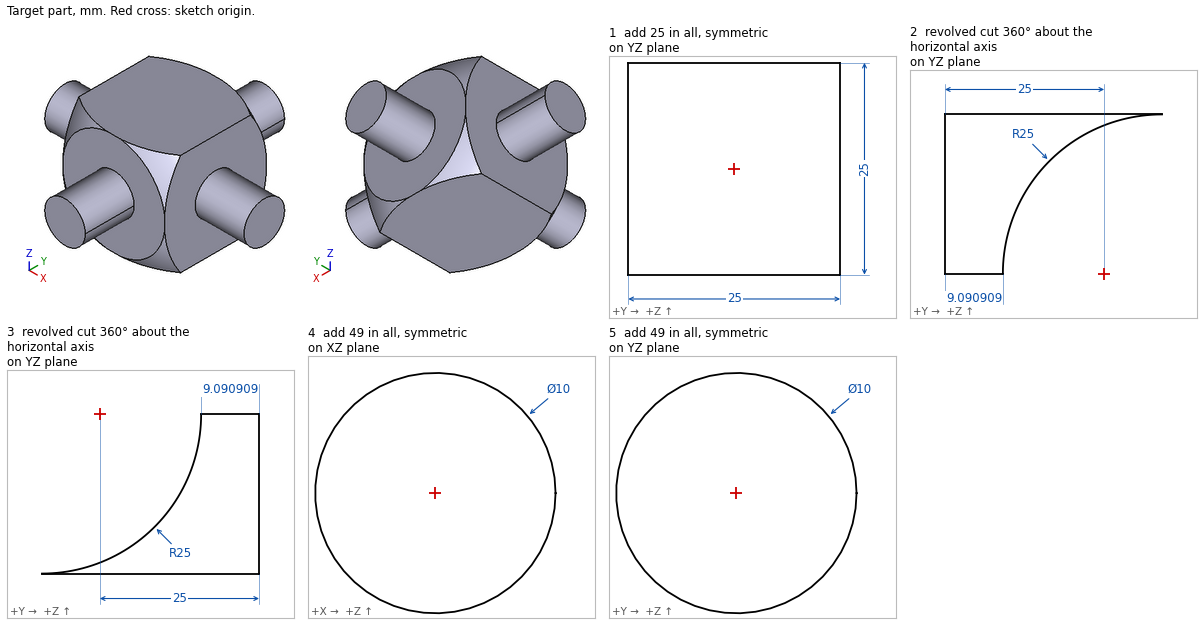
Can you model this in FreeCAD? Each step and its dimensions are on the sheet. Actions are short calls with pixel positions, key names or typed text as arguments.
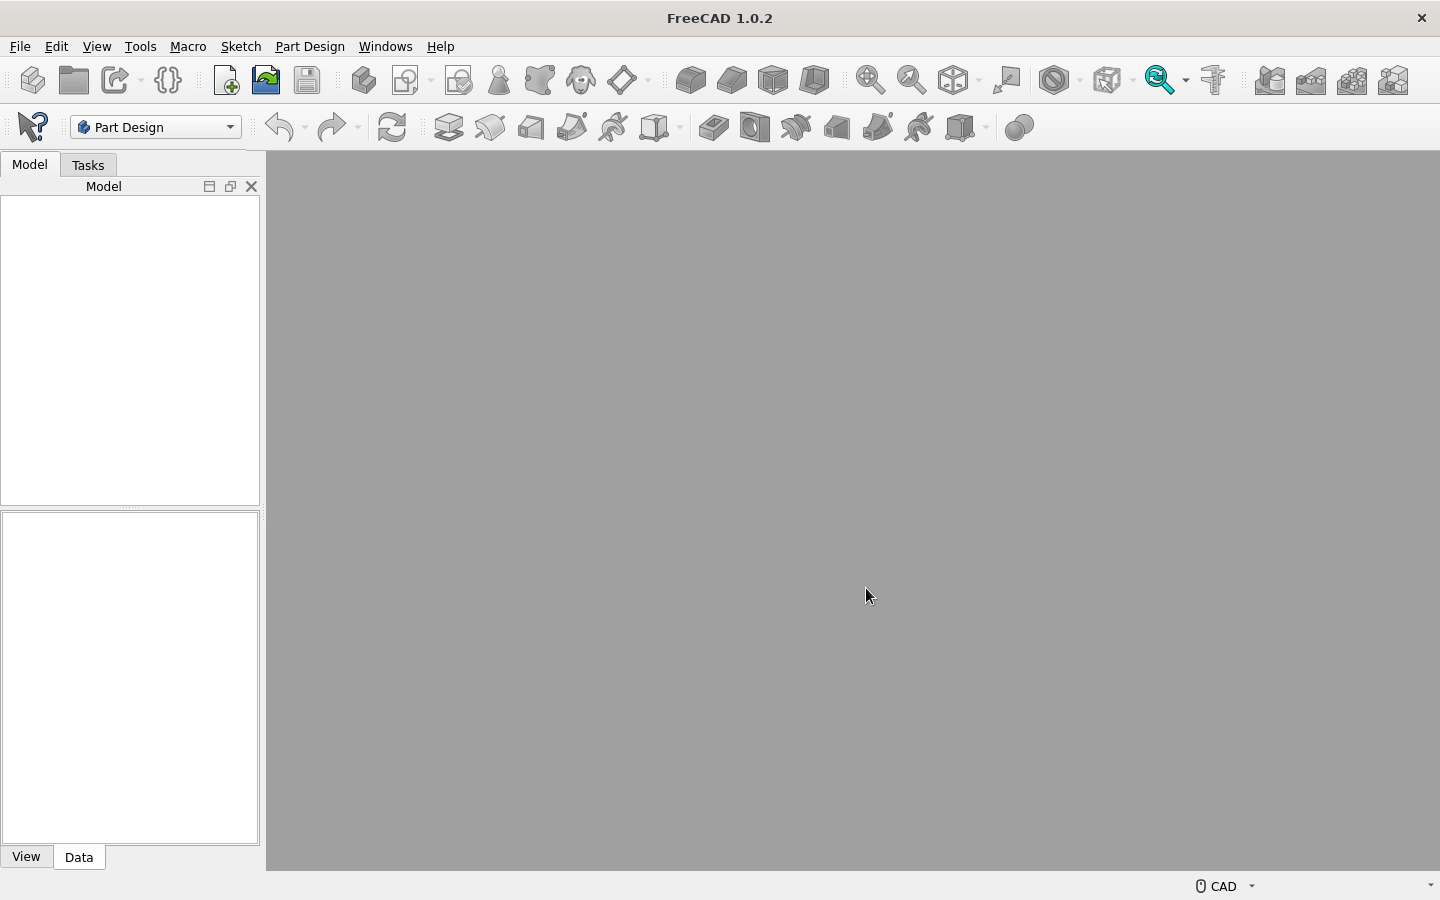
key(ctrl+n)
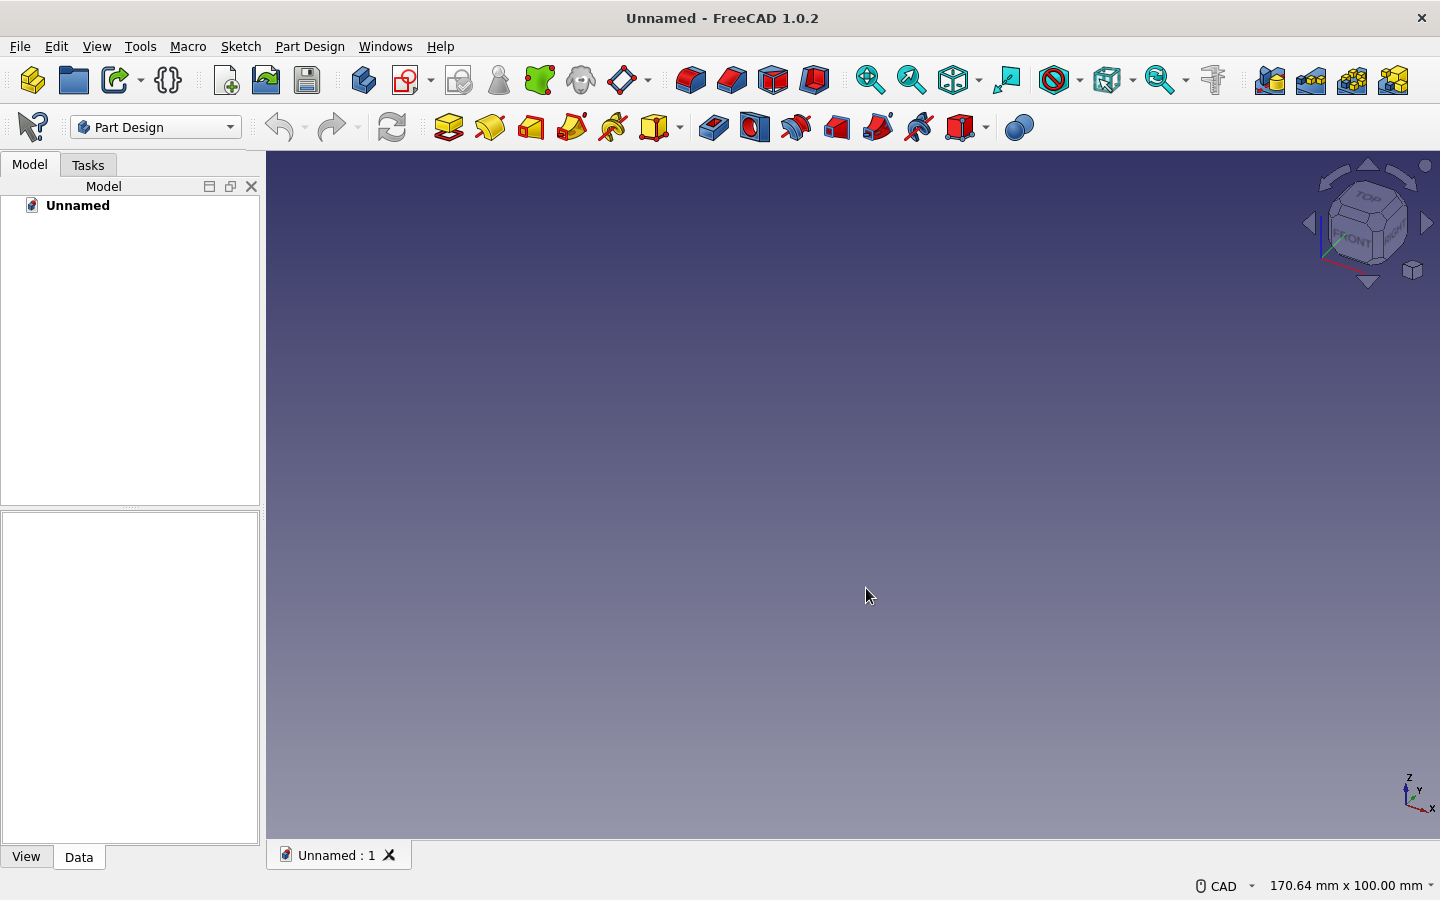
click(404, 80)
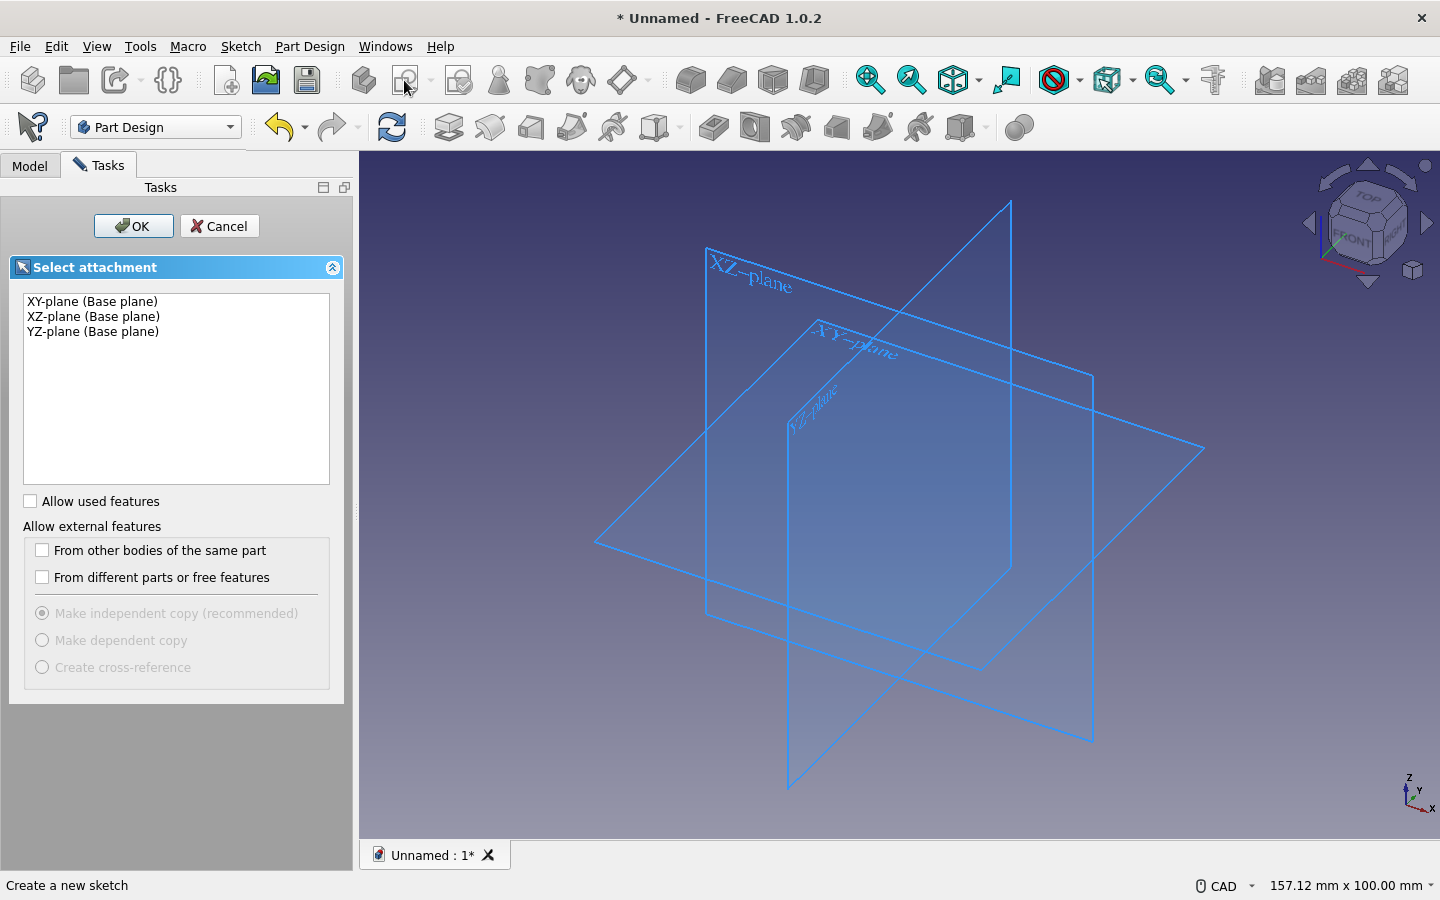
click(84, 332)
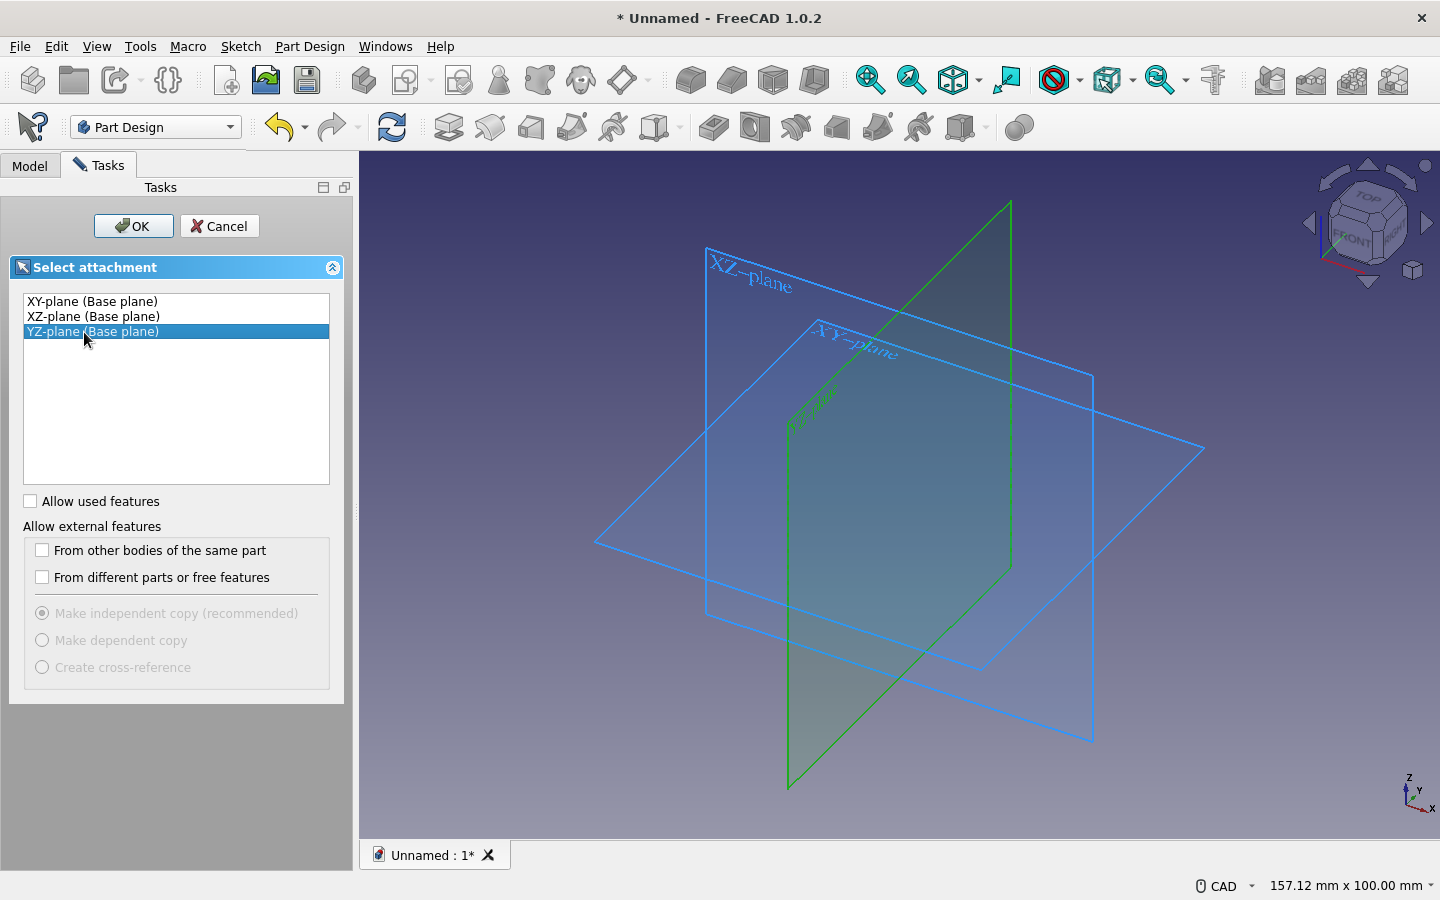
click(134, 226)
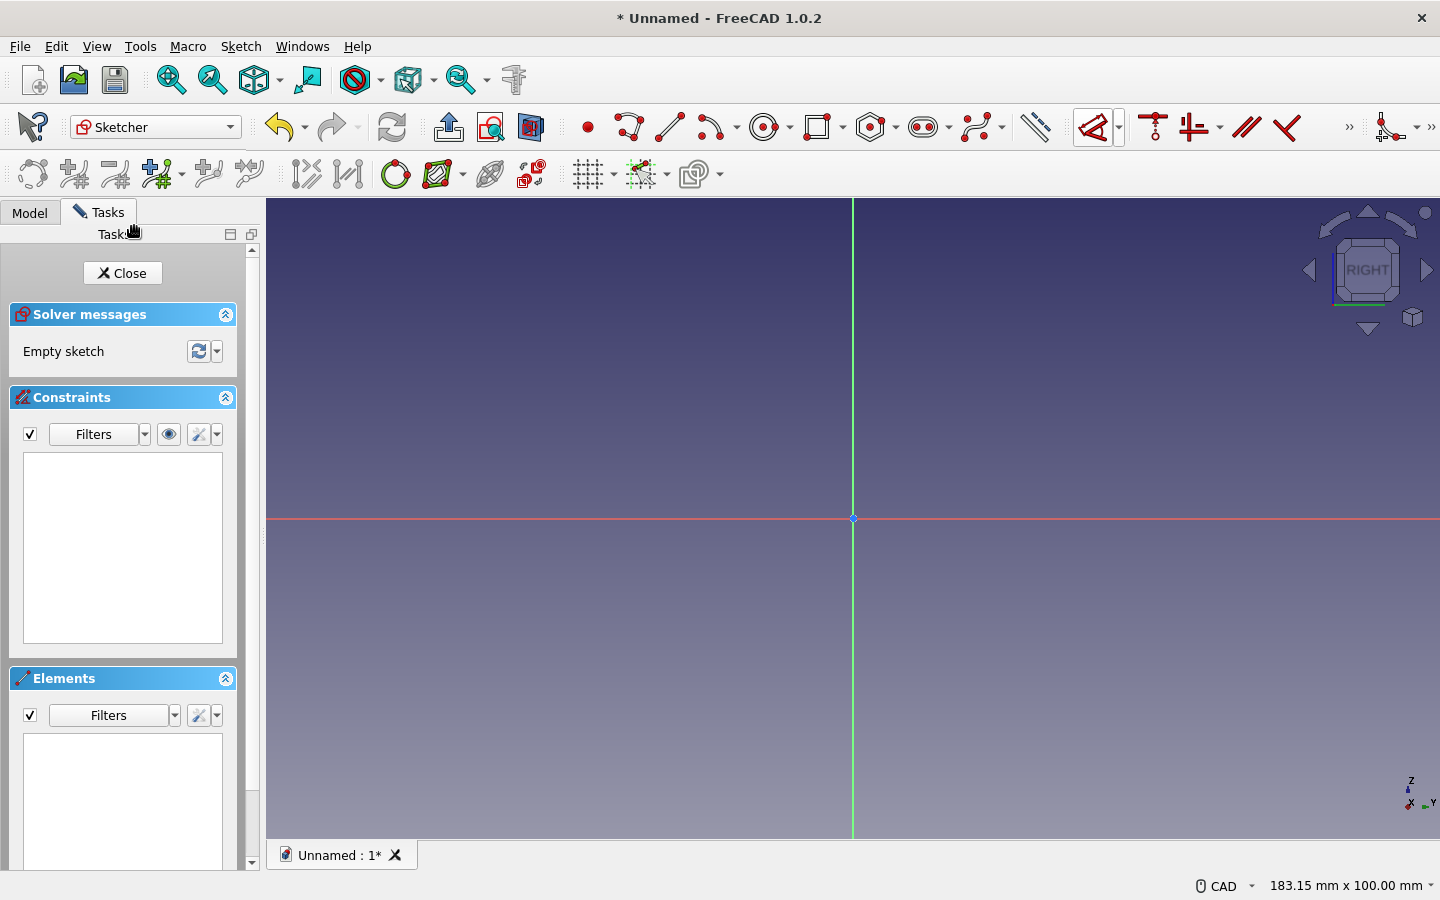
scroll(893, 518, up, 5)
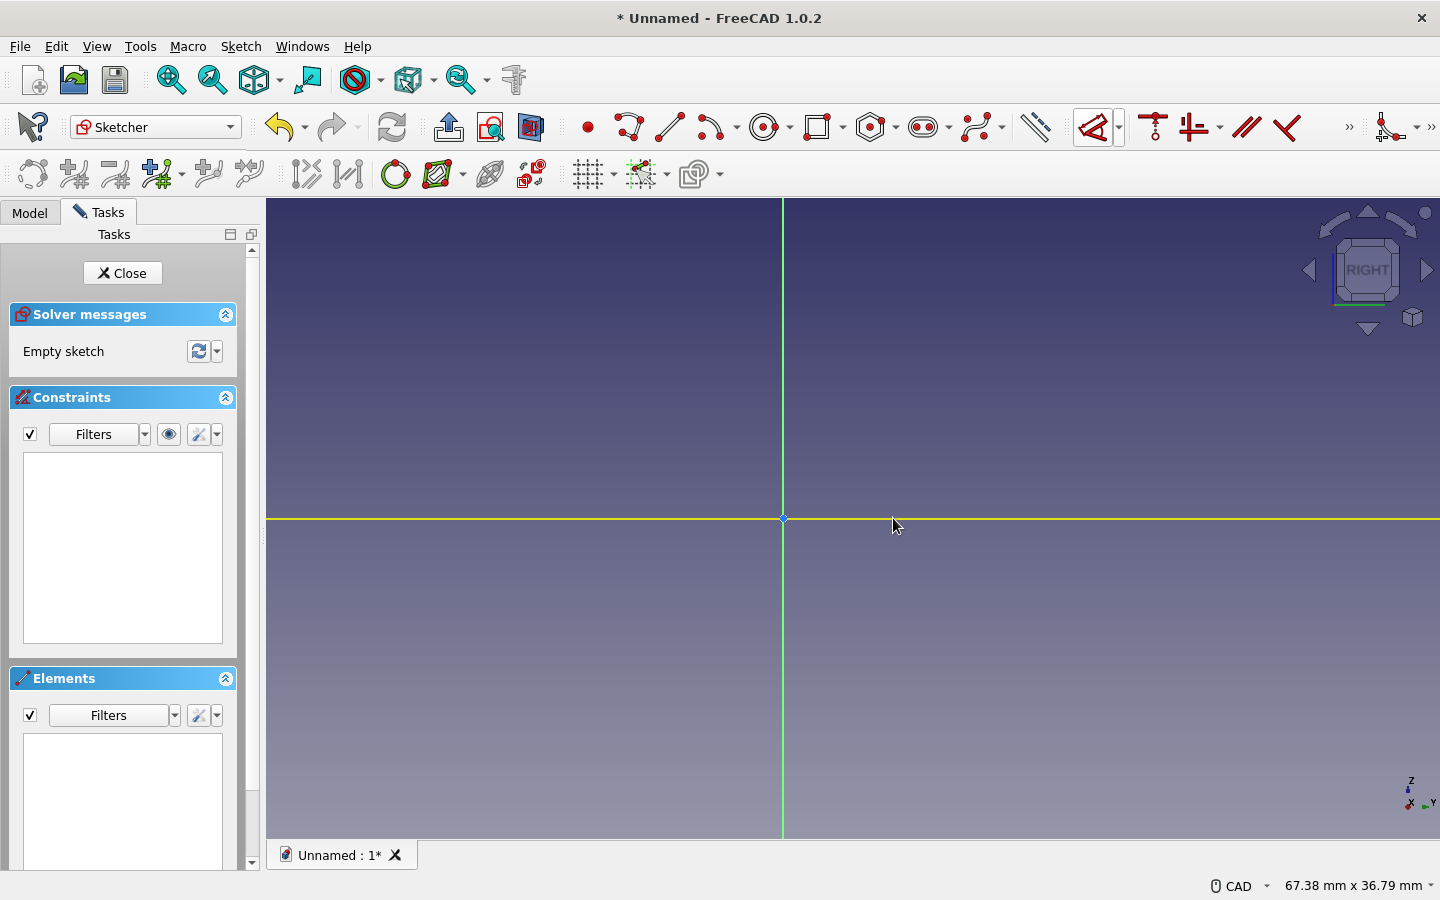
key(g)
key(v)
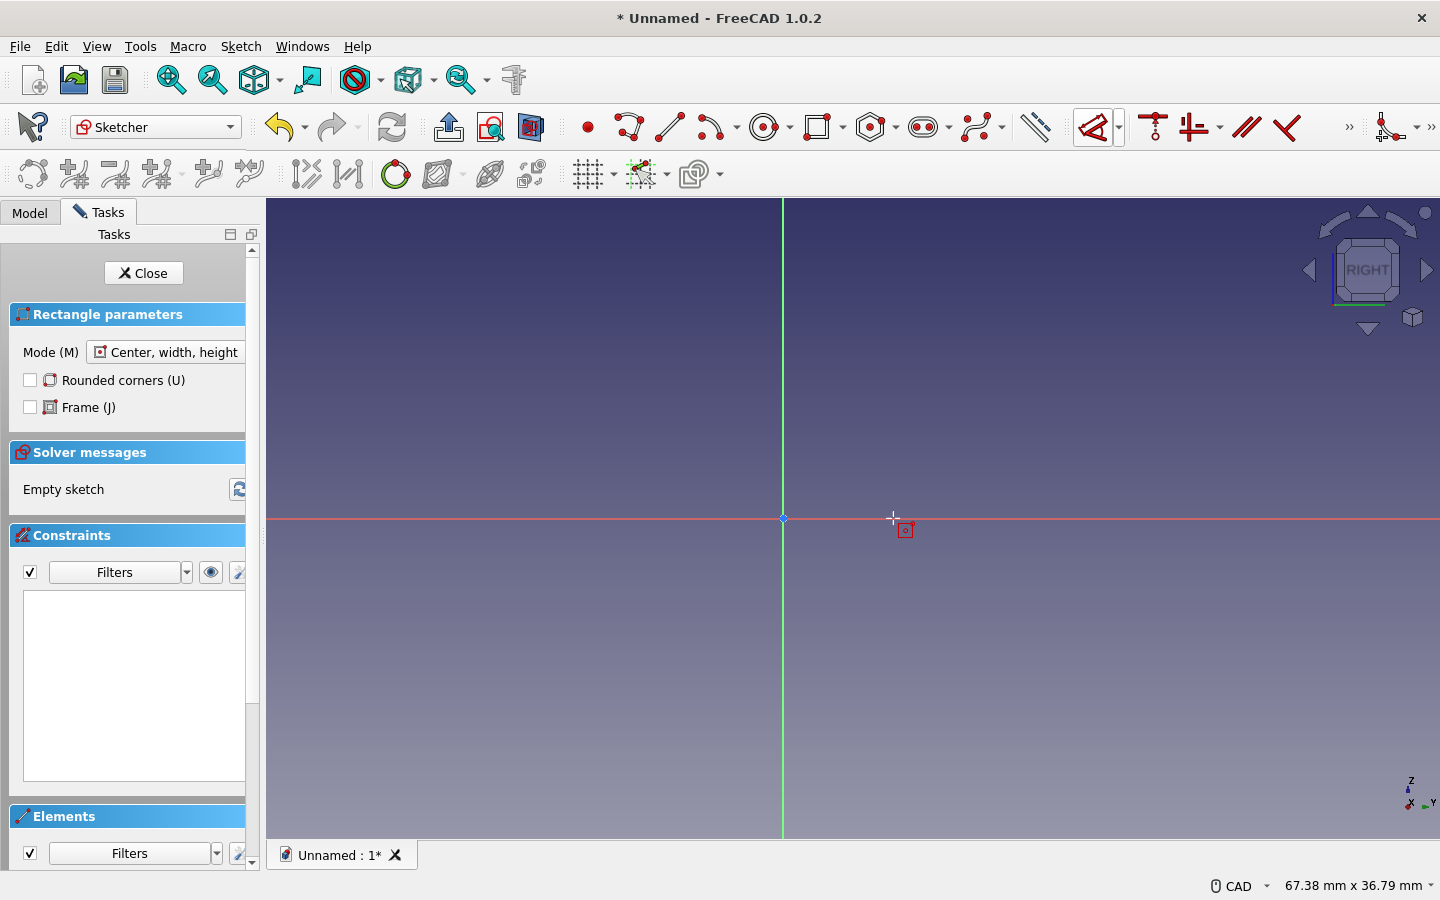
click(783, 518)
click(1001, 301)
key(Escape)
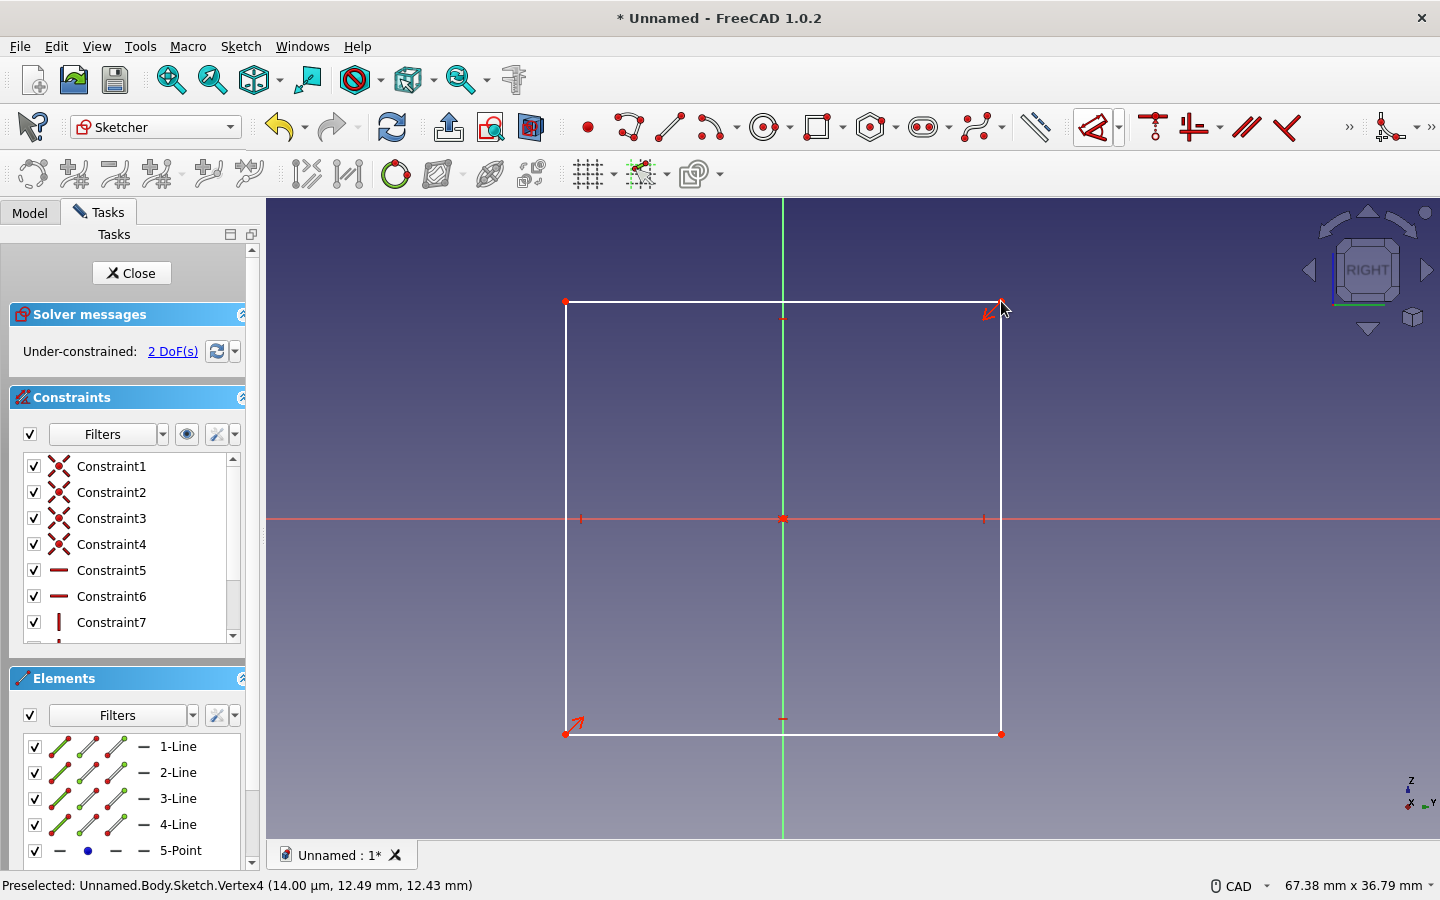
key(d)